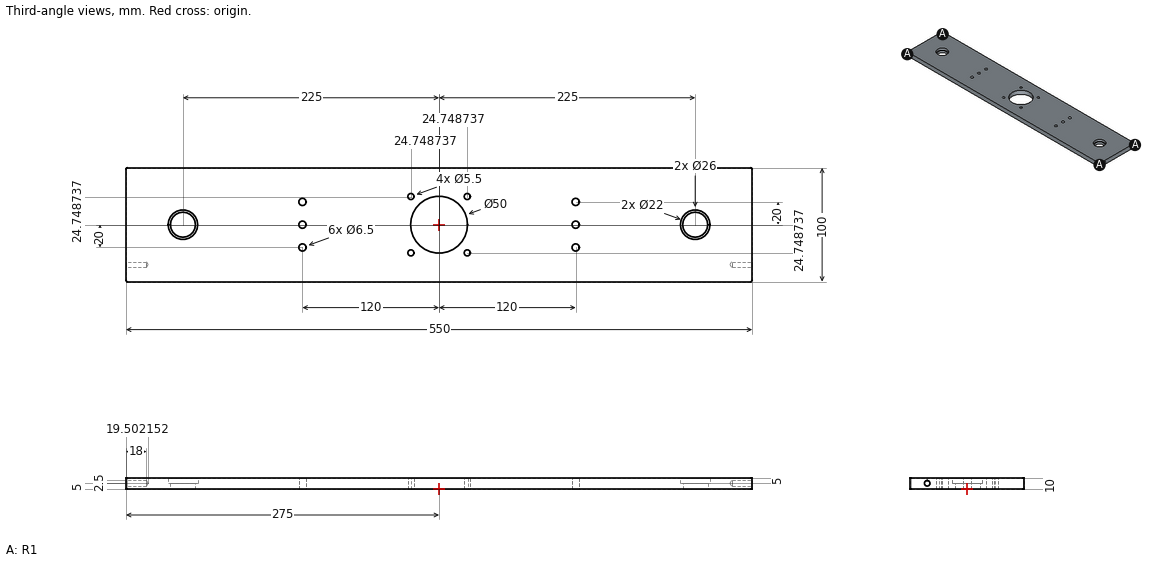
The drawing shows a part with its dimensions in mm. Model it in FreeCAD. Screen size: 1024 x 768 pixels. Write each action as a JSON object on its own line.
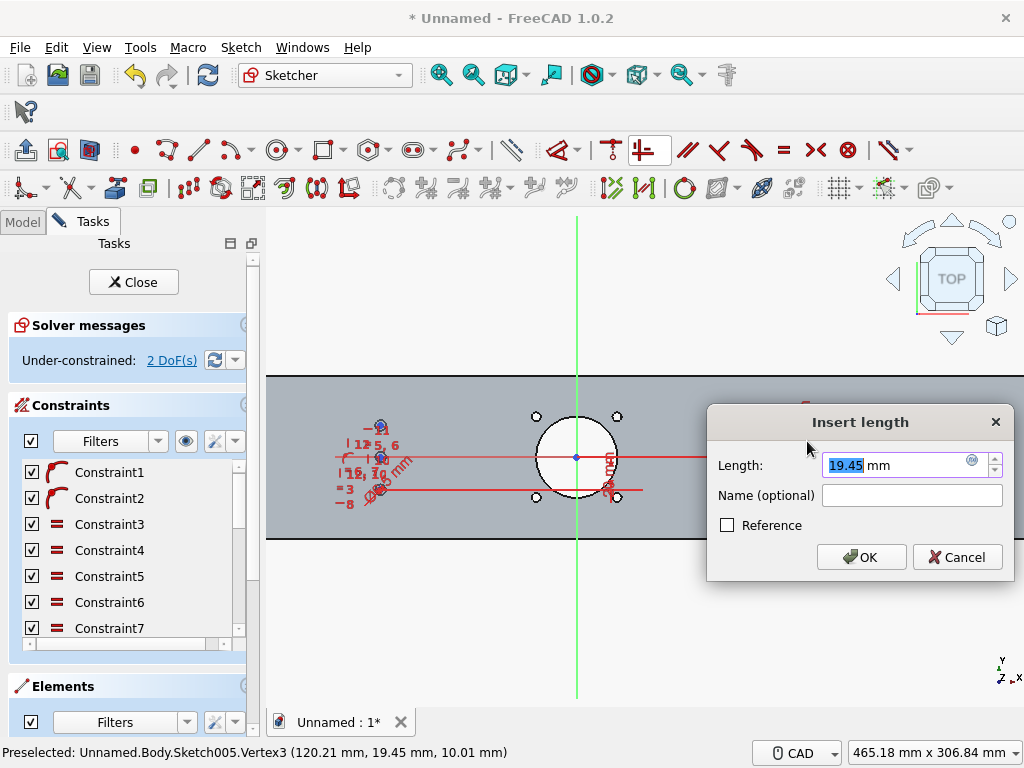
{"action": "type", "text": "20"}
{"action": "key", "text": "Return"}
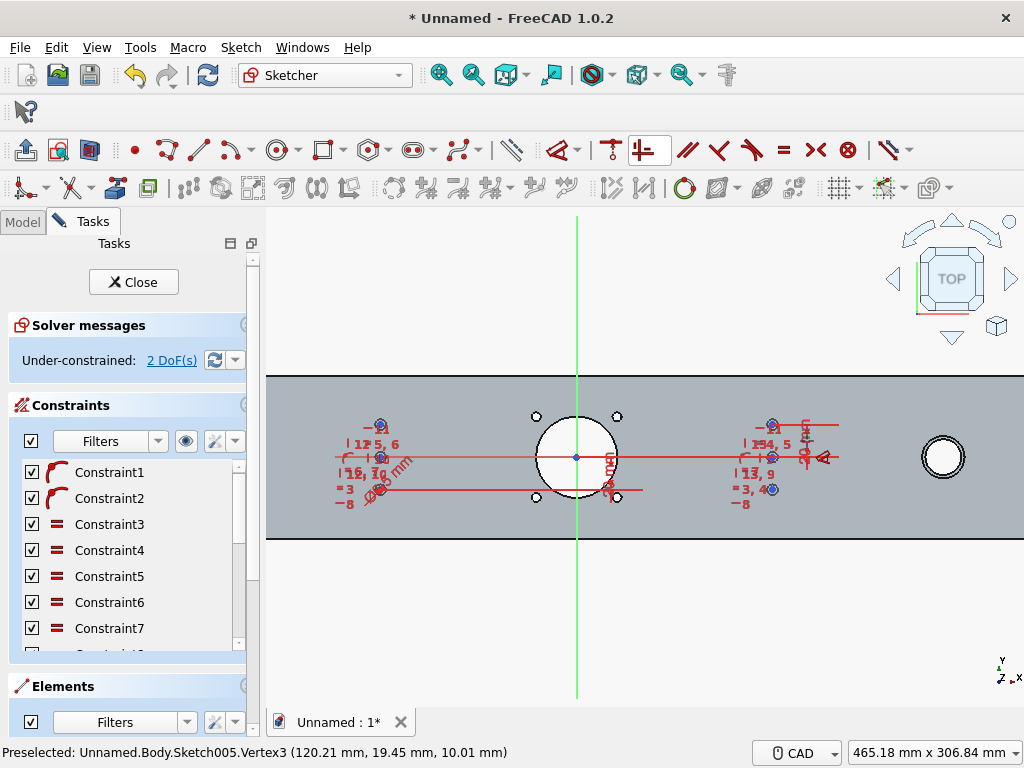
{"action": "left_click", "coordinate": [381, 490]}
{"action": "left_click", "coordinate": [479, 524]}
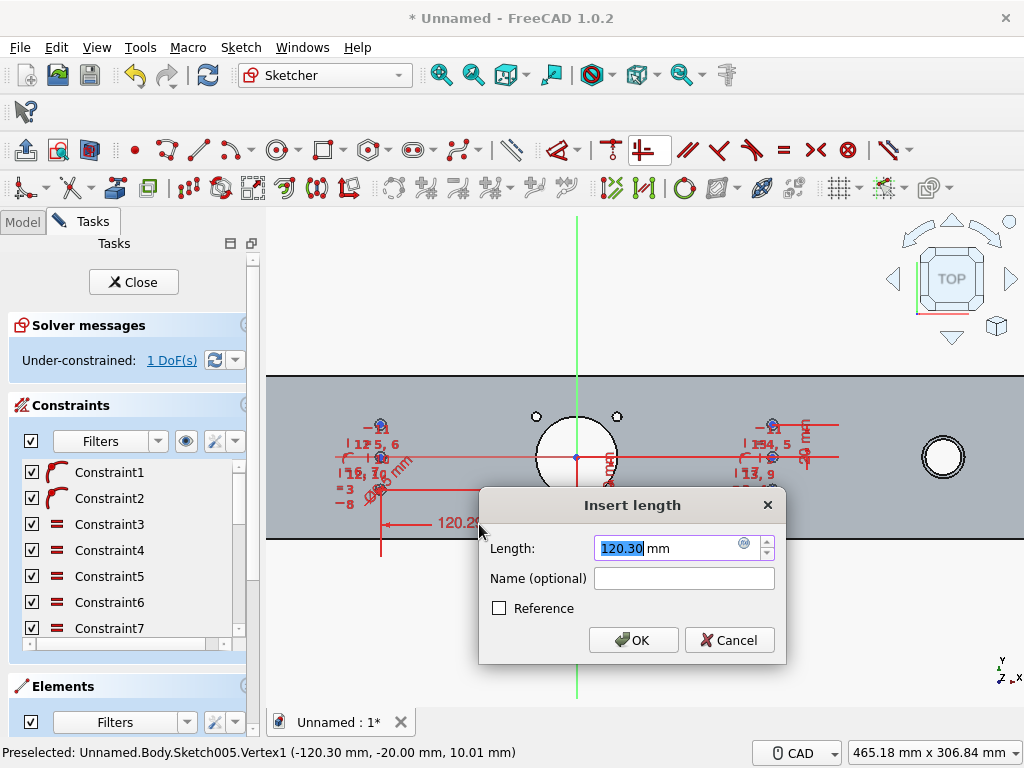
{"action": "type", "text": "120"}
{"action": "key", "text": "Return"}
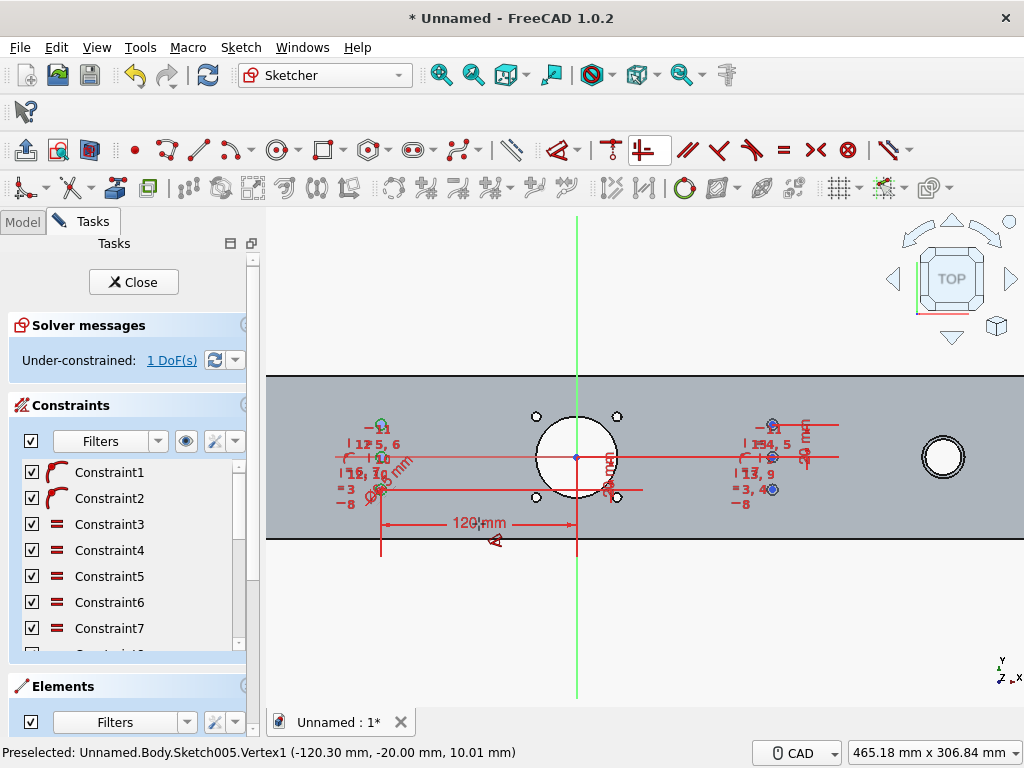
{"action": "left_click", "coordinate": [773, 490]}
{"action": "left_click", "coordinate": [675, 524]}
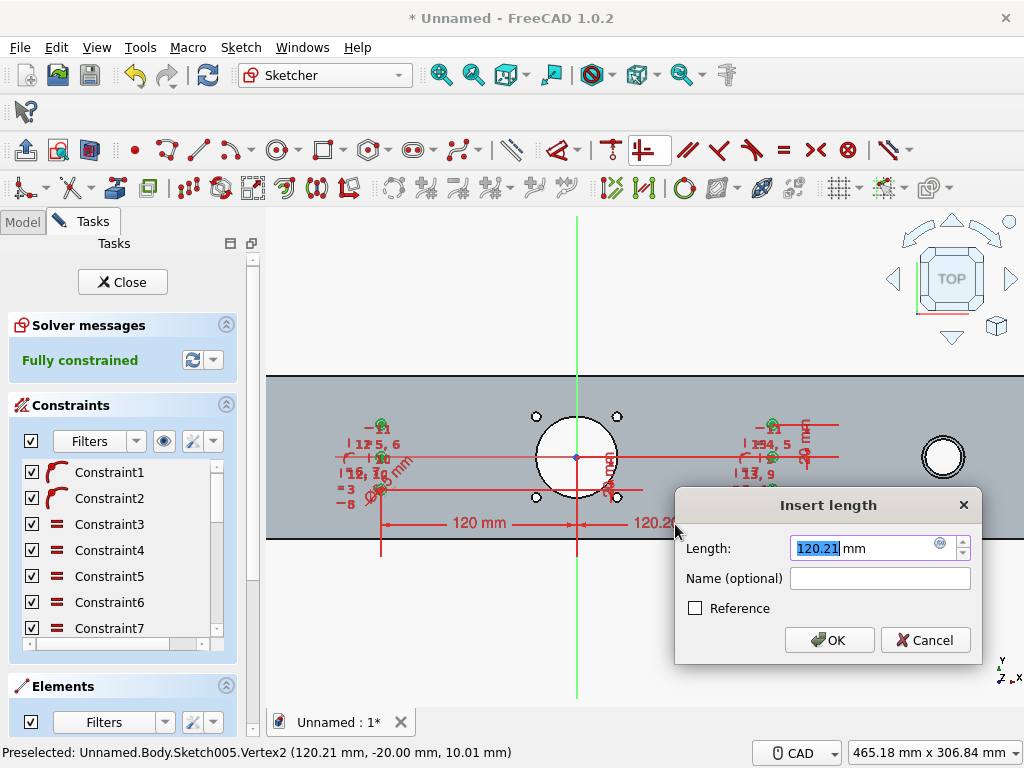
{"action": "type", "text": "120"}
{"action": "key", "text": "Return"}
{"action": "key", "text": "Escape"}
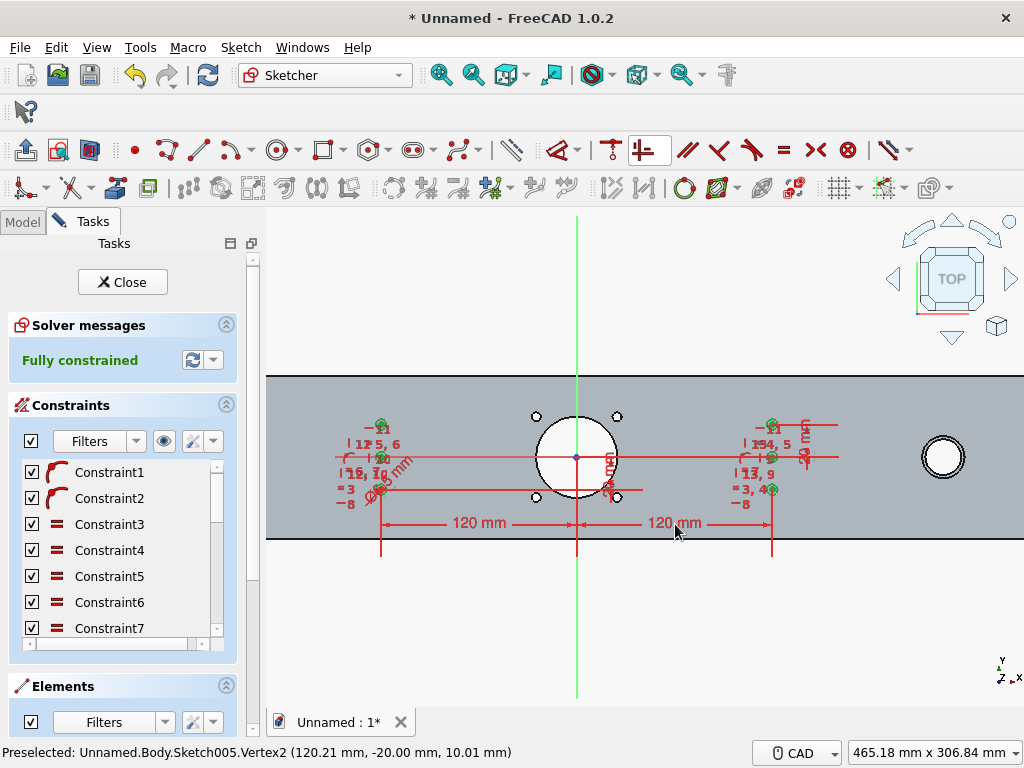
{"action": "left_click", "coordinate": [123, 282]}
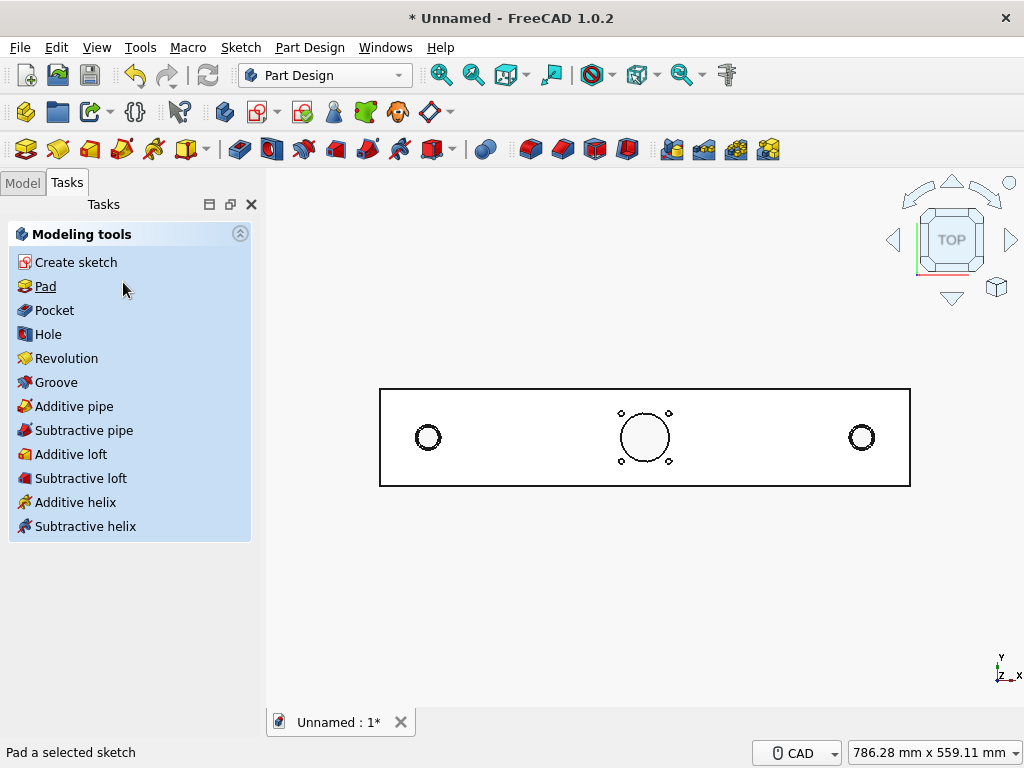
{"action": "left_click", "coordinate": [240, 150]}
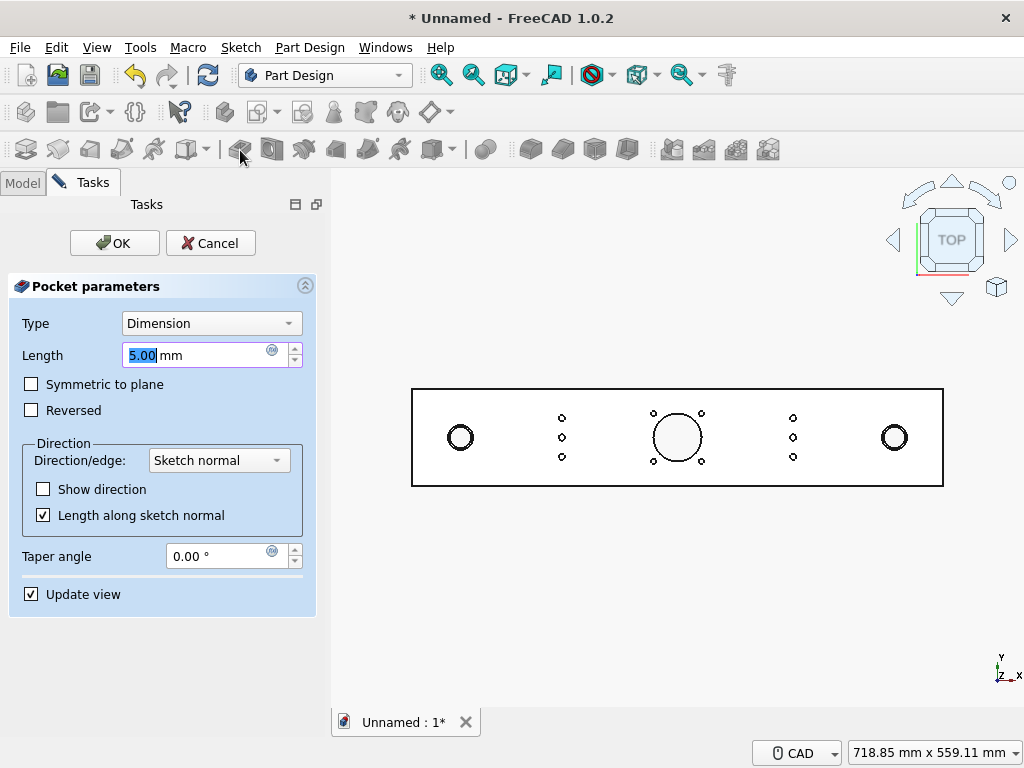
{"action": "left_click", "coordinate": [212, 324]}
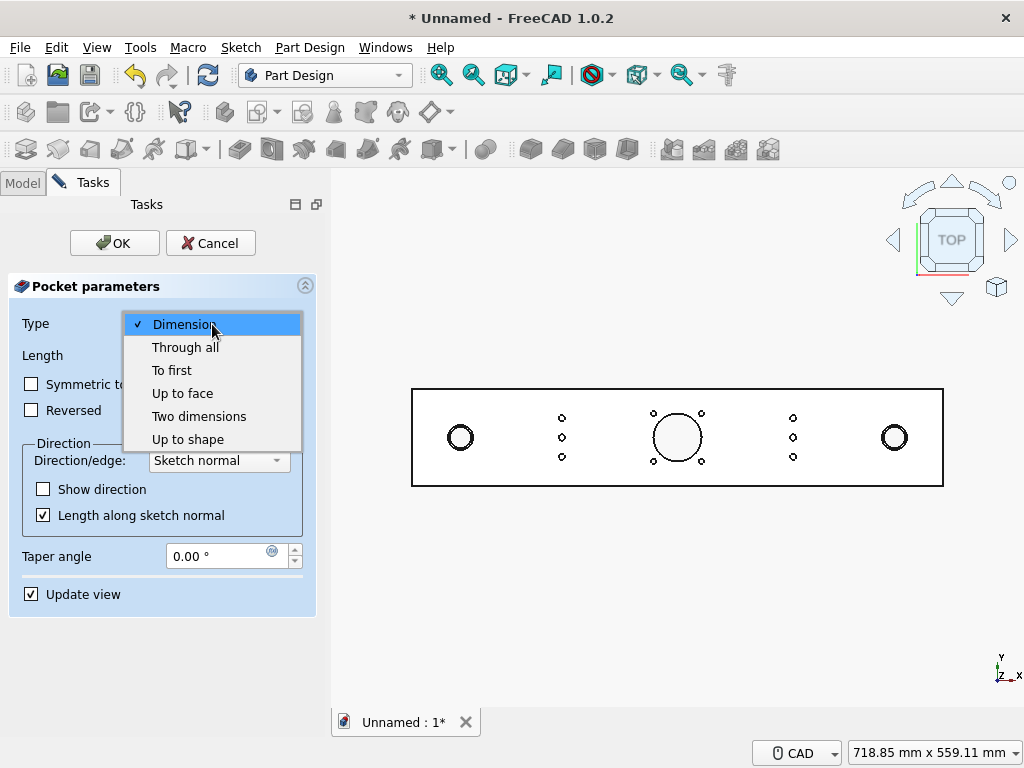
{"action": "left_click", "coordinate": [212, 348]}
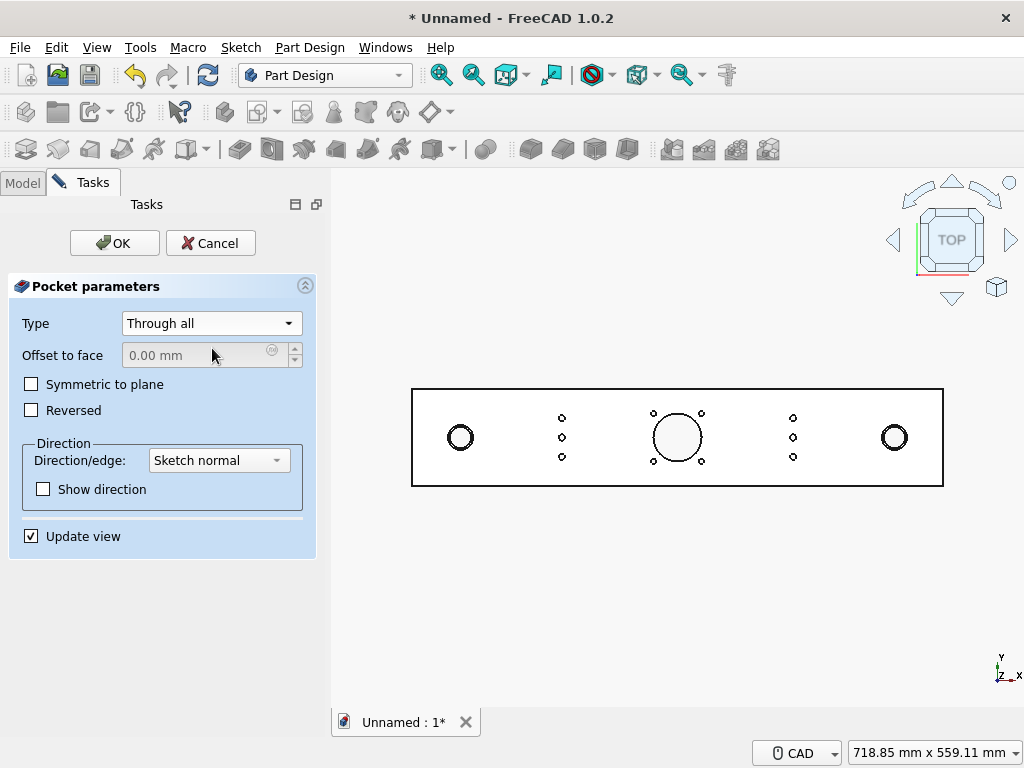
{"action": "left_click", "coordinate": [115, 243]}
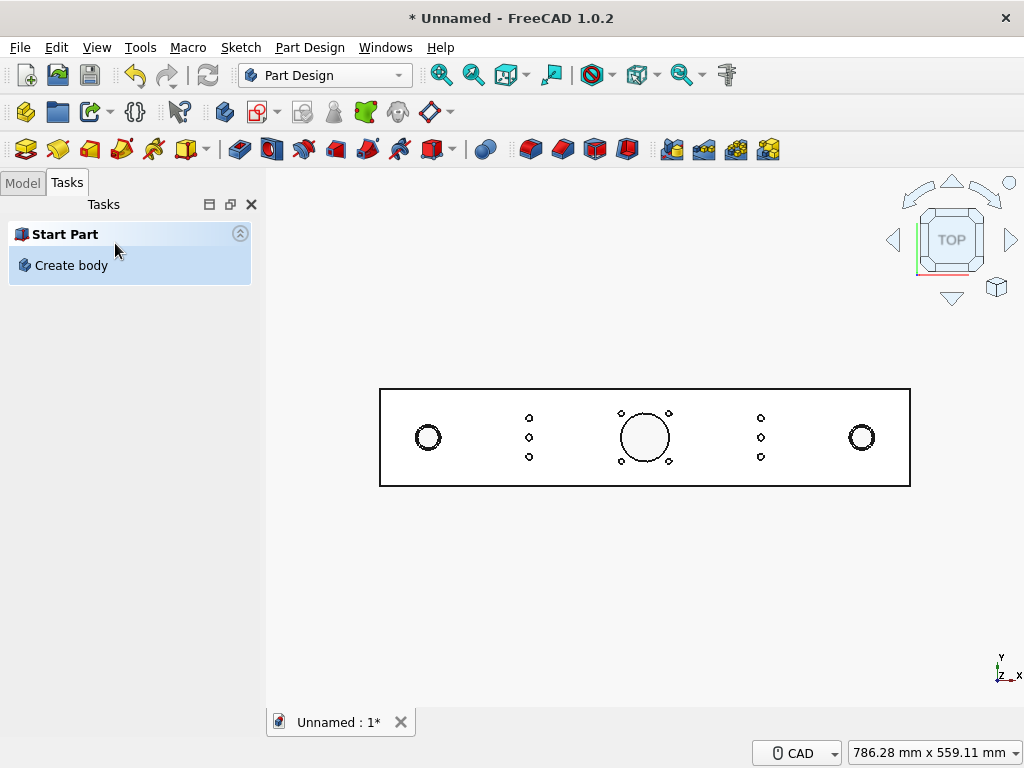
{"action": "scroll", "coordinate": [380, 388], "scroll_direction": "up", "scroll_amount": 8}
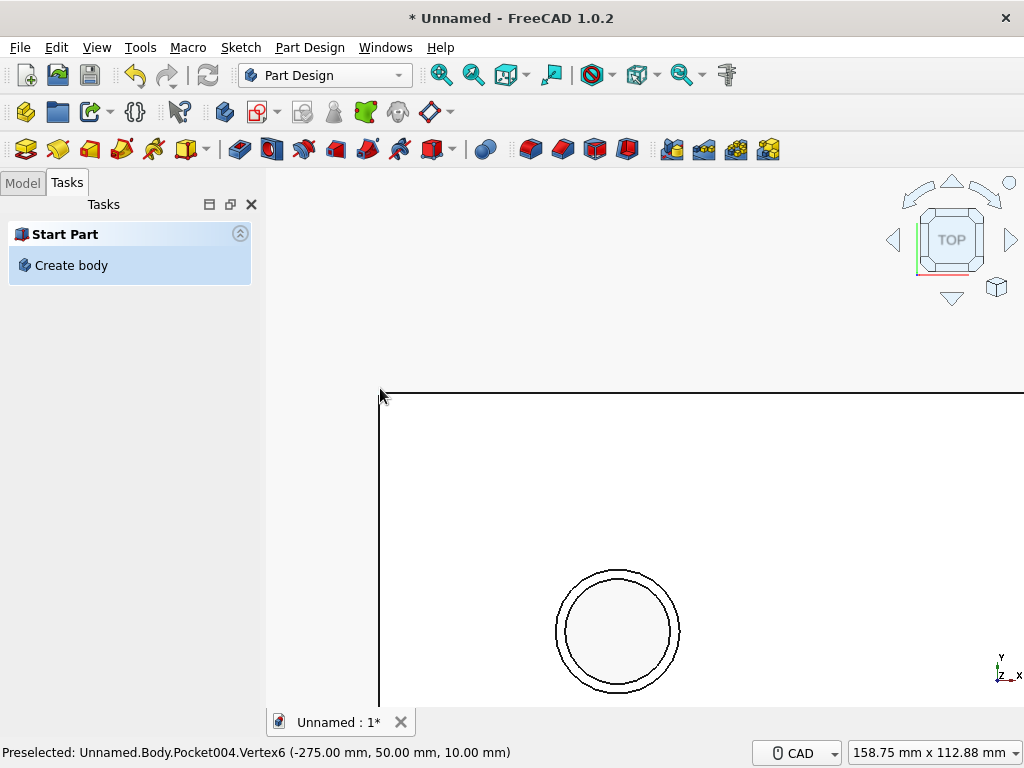
{"action": "key", "text": "v f"}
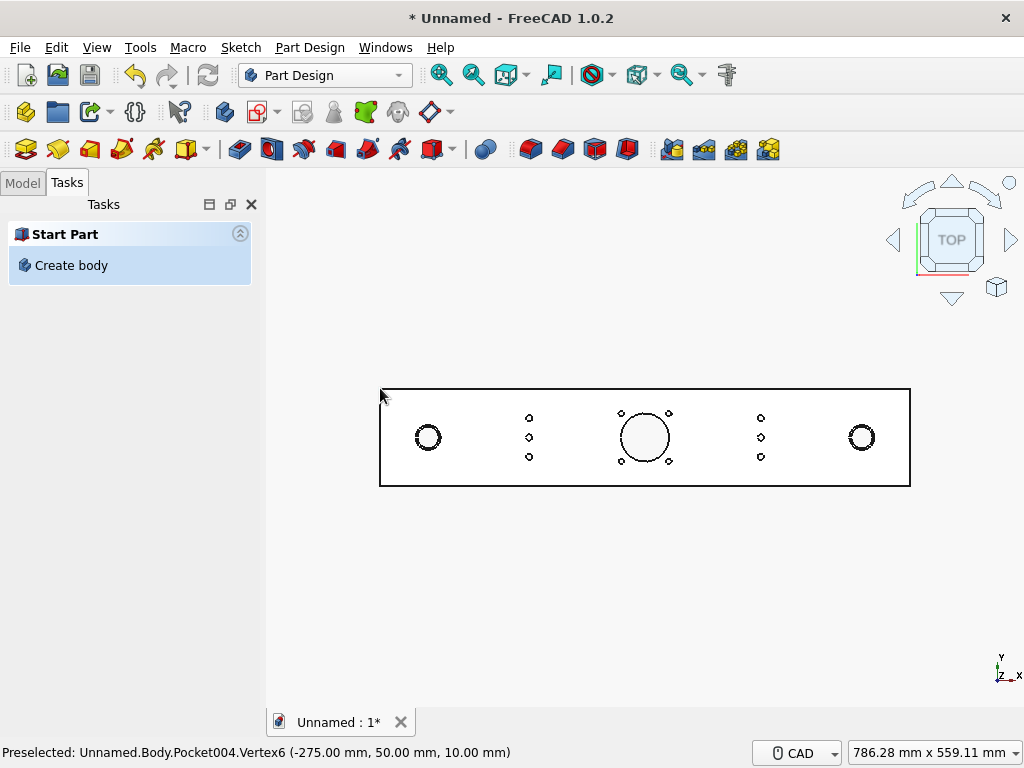
{"action": "key", "text": "0"}